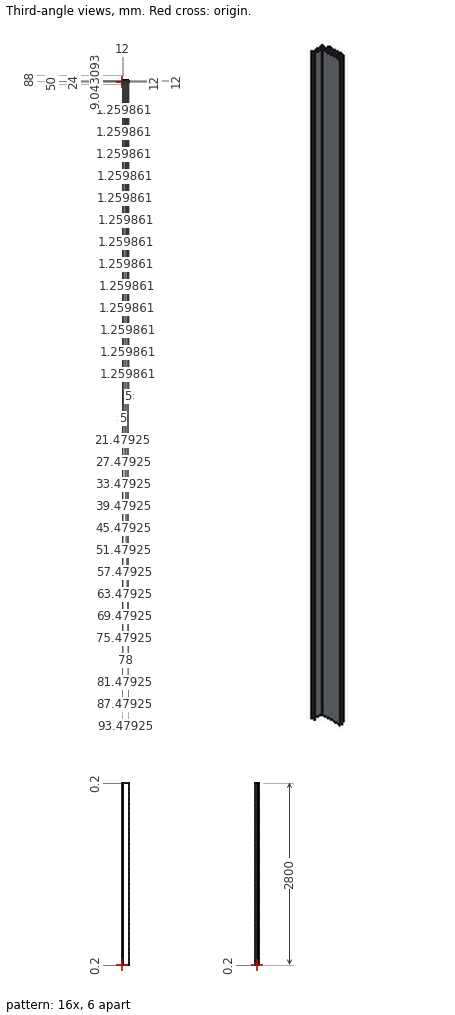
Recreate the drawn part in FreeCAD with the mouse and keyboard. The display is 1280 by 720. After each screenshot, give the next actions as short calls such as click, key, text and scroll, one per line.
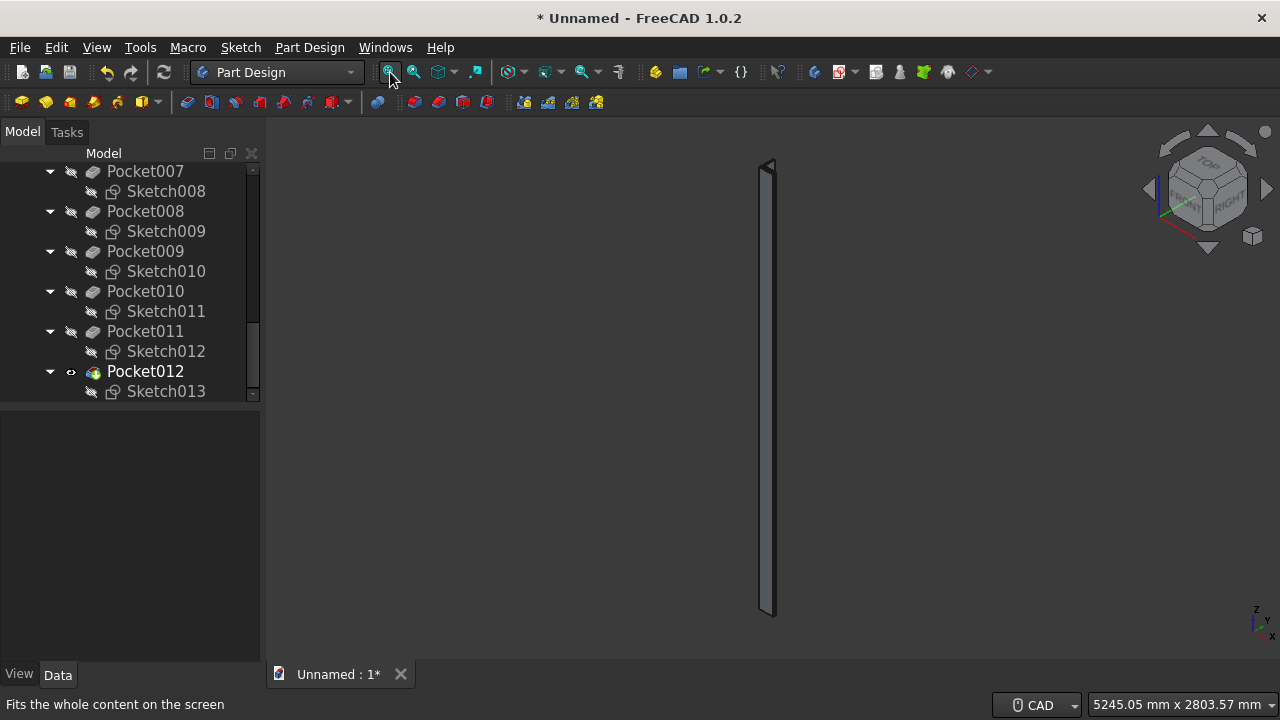
scroll(771, 172, up, 11)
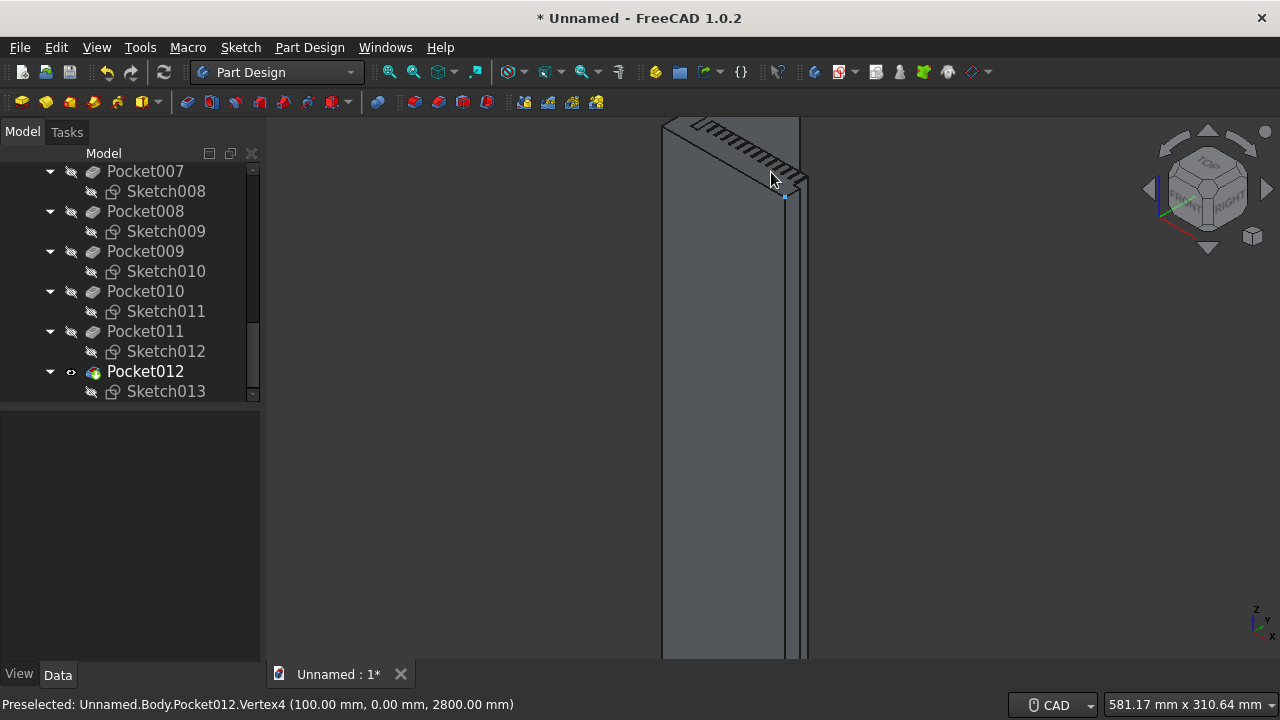
click(390, 72)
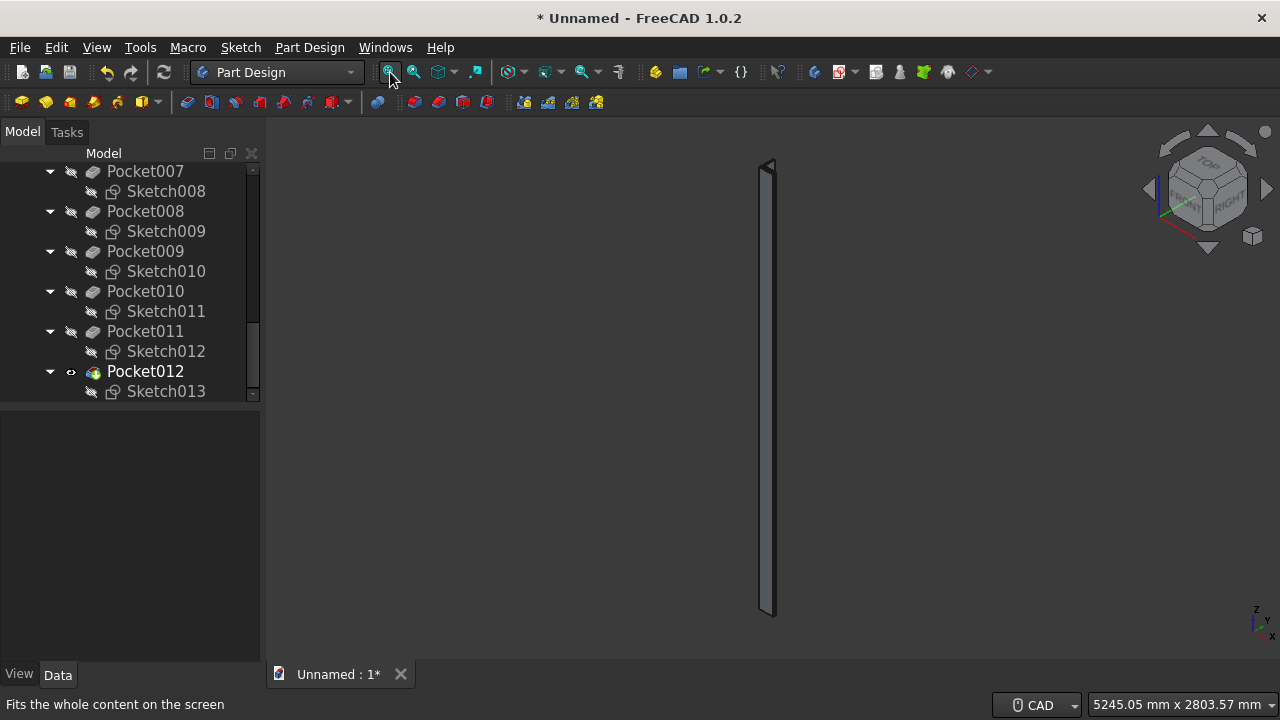
key(2)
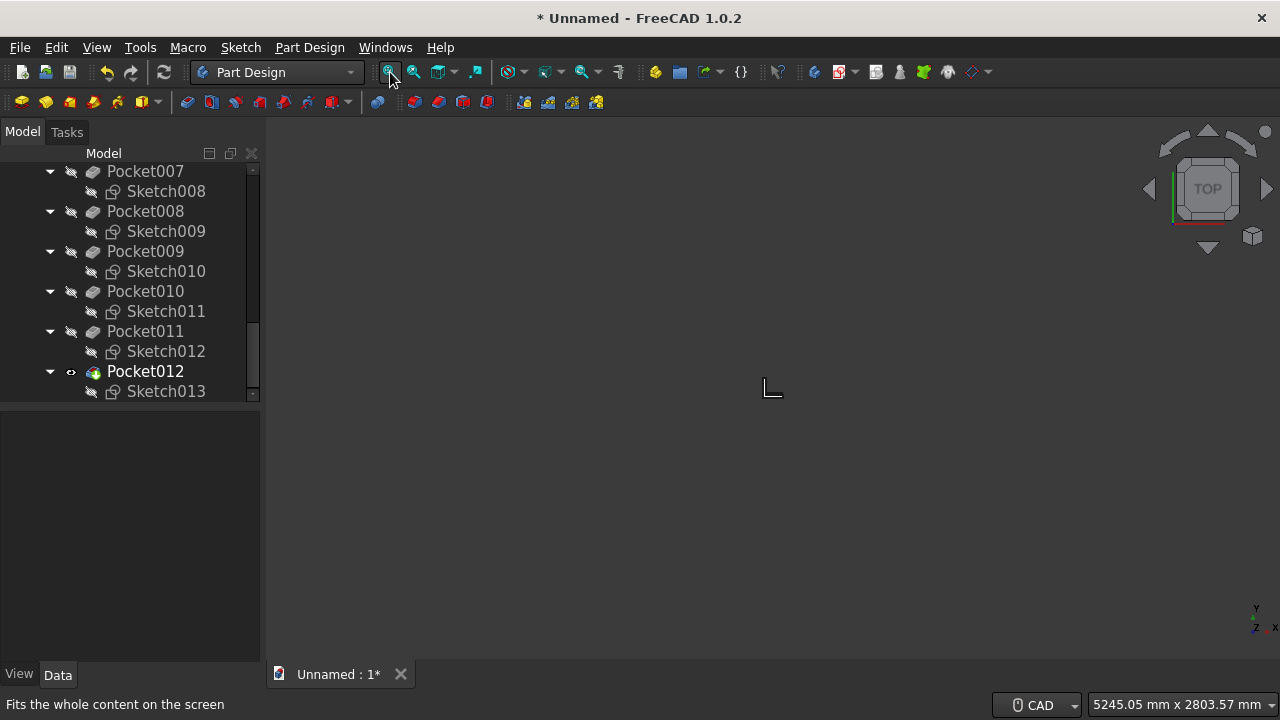
click(390, 72)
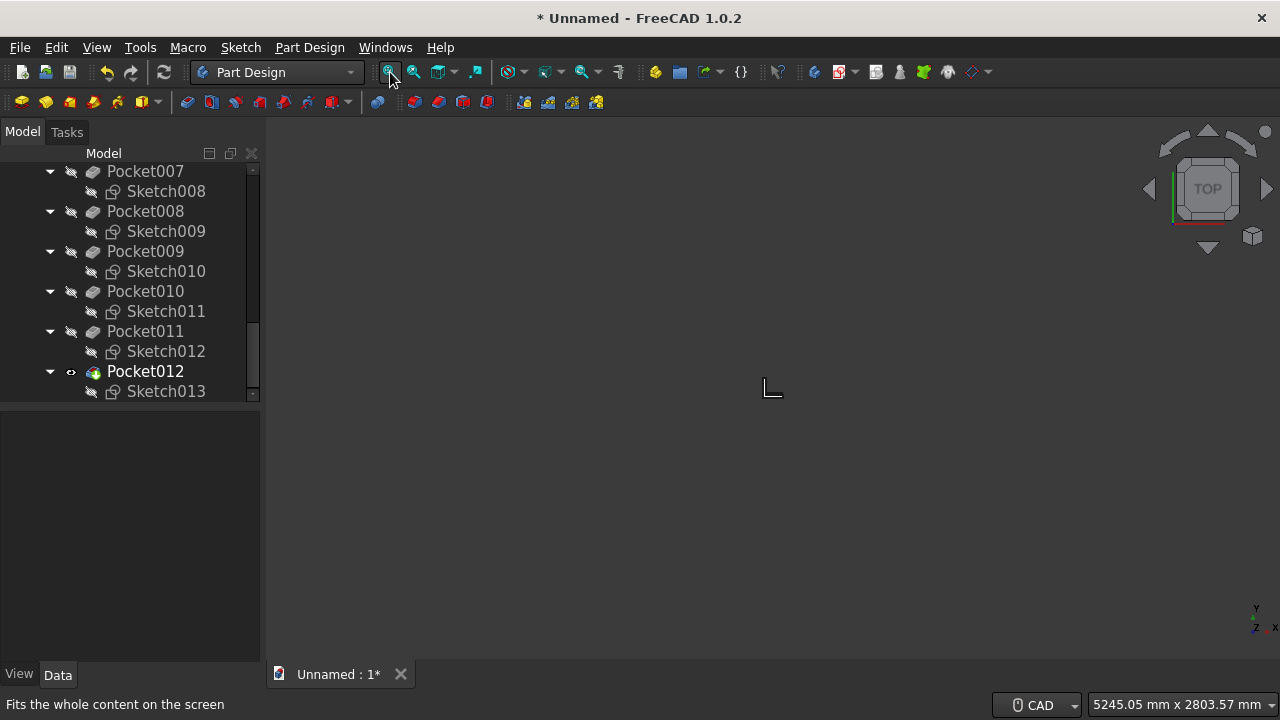
scroll(779, 395, up, 11)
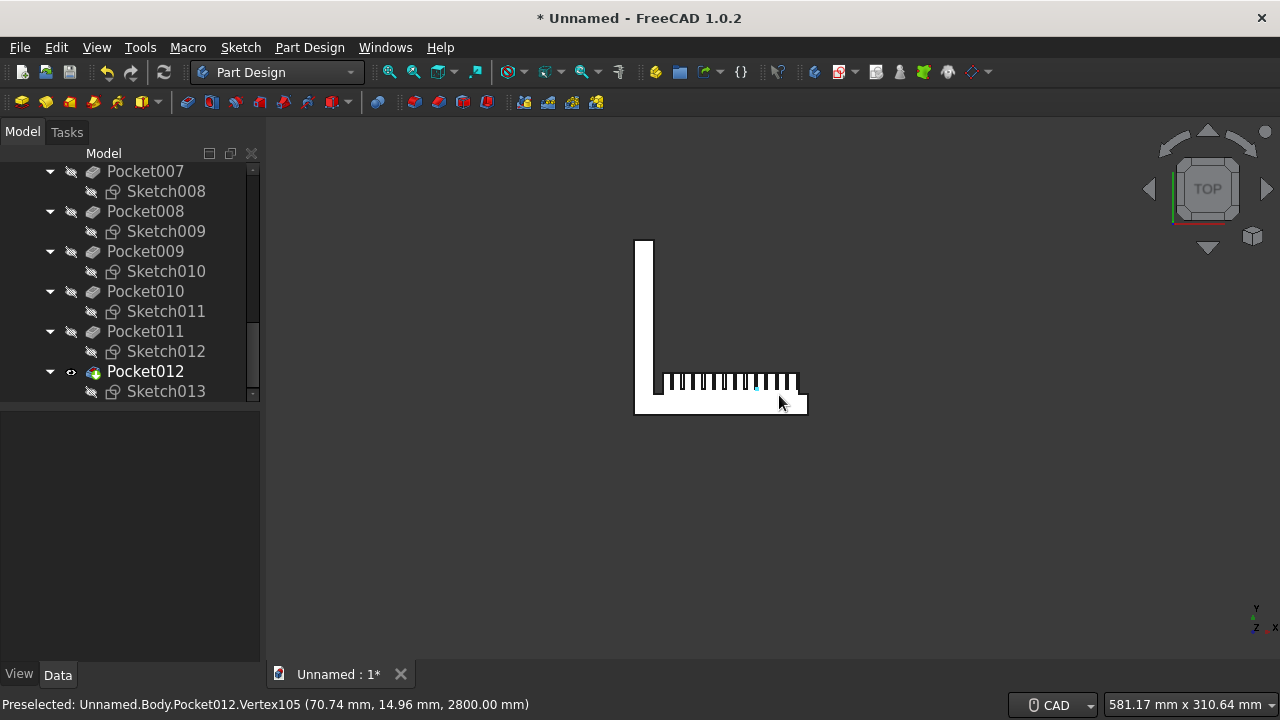
click(771, 401)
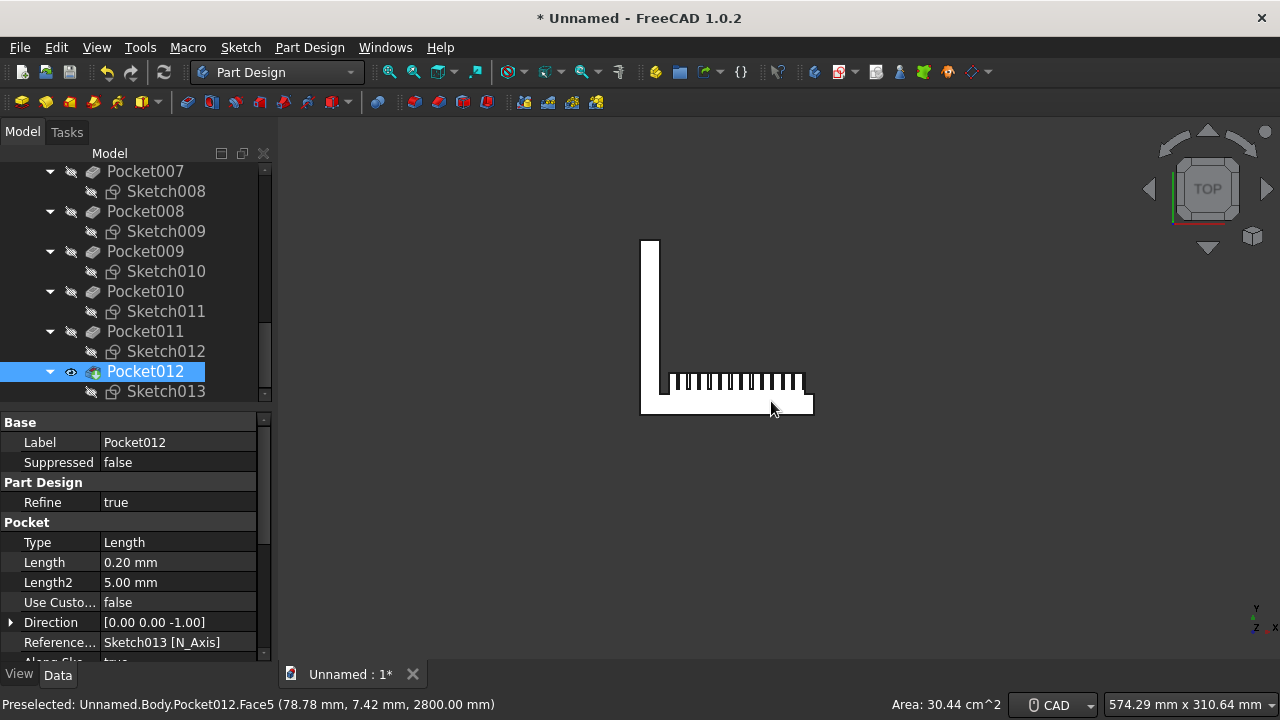
click(840, 72)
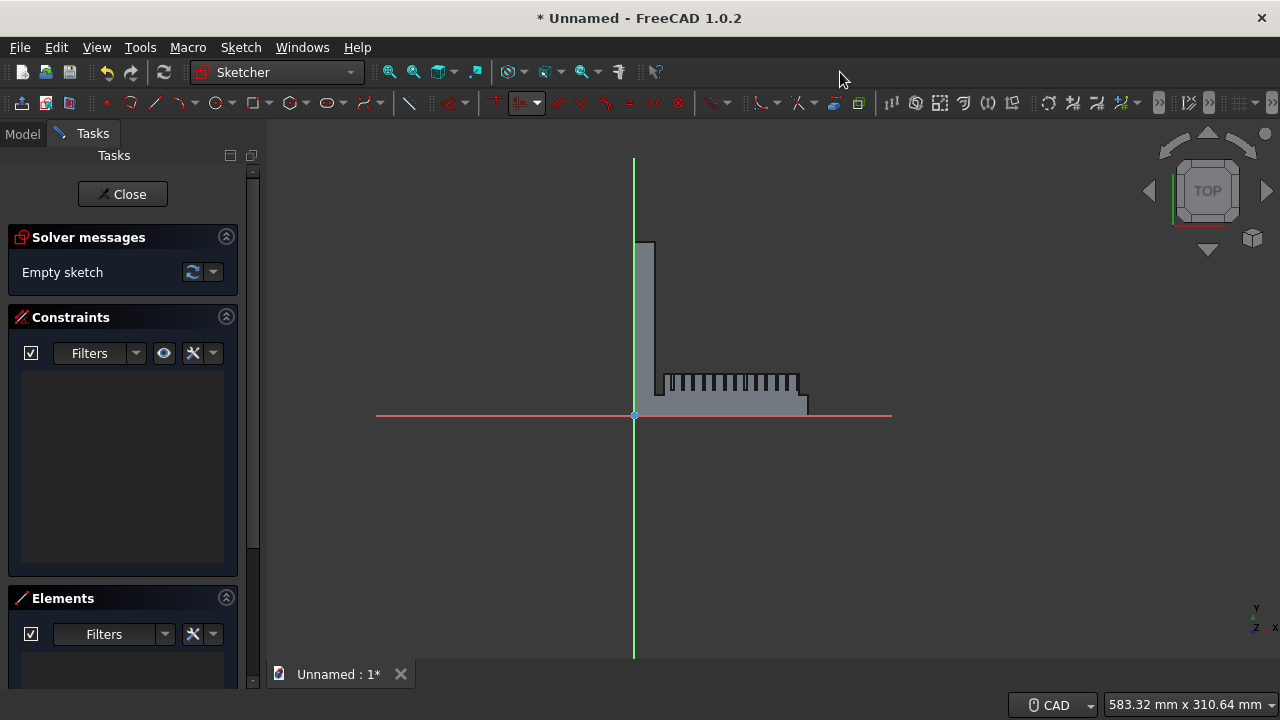
scroll(625, 455, up, 7)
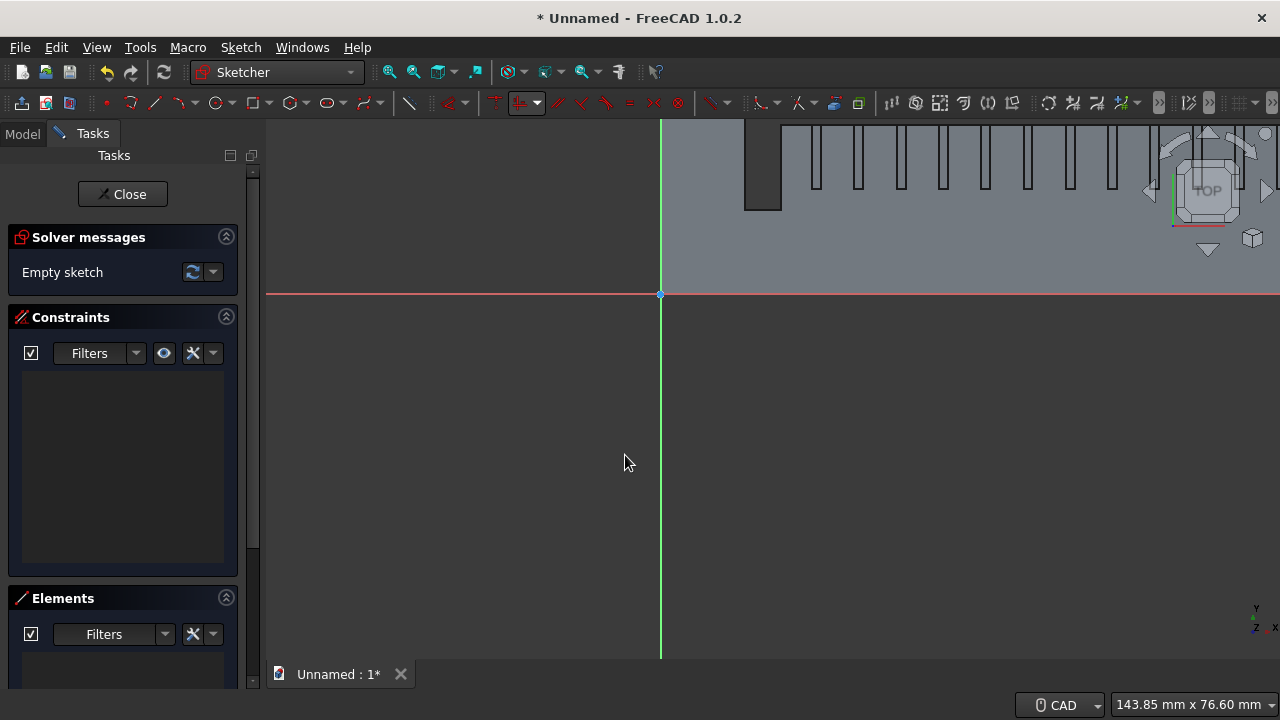
click(254, 104)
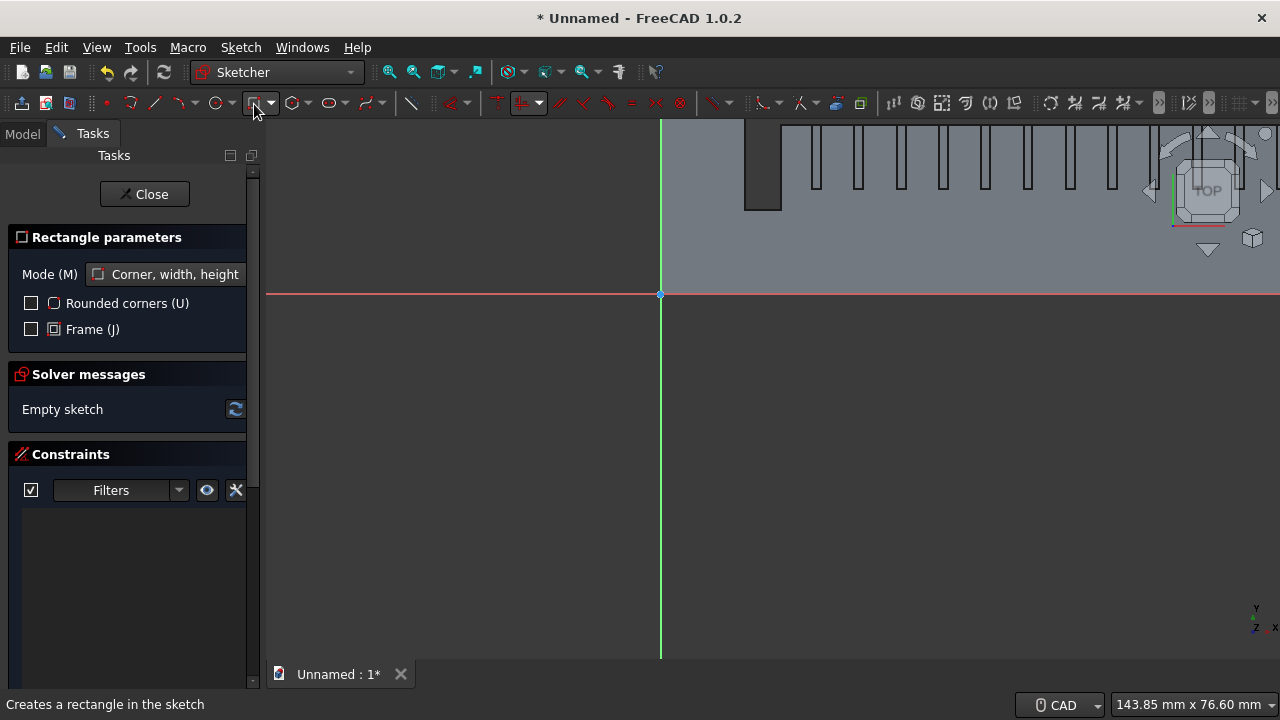
click(661, 210)
move(745, 562)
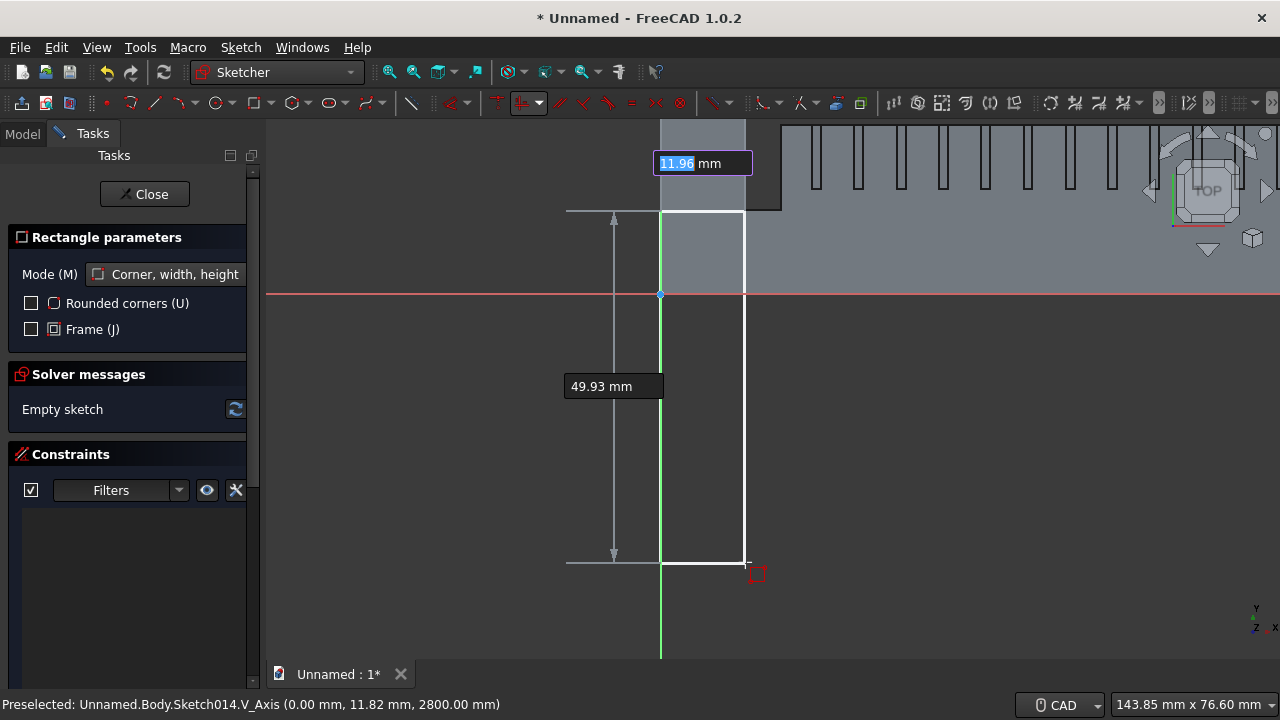
text(12)
key(Tab)
text(50)
key(Return)
key(Escape)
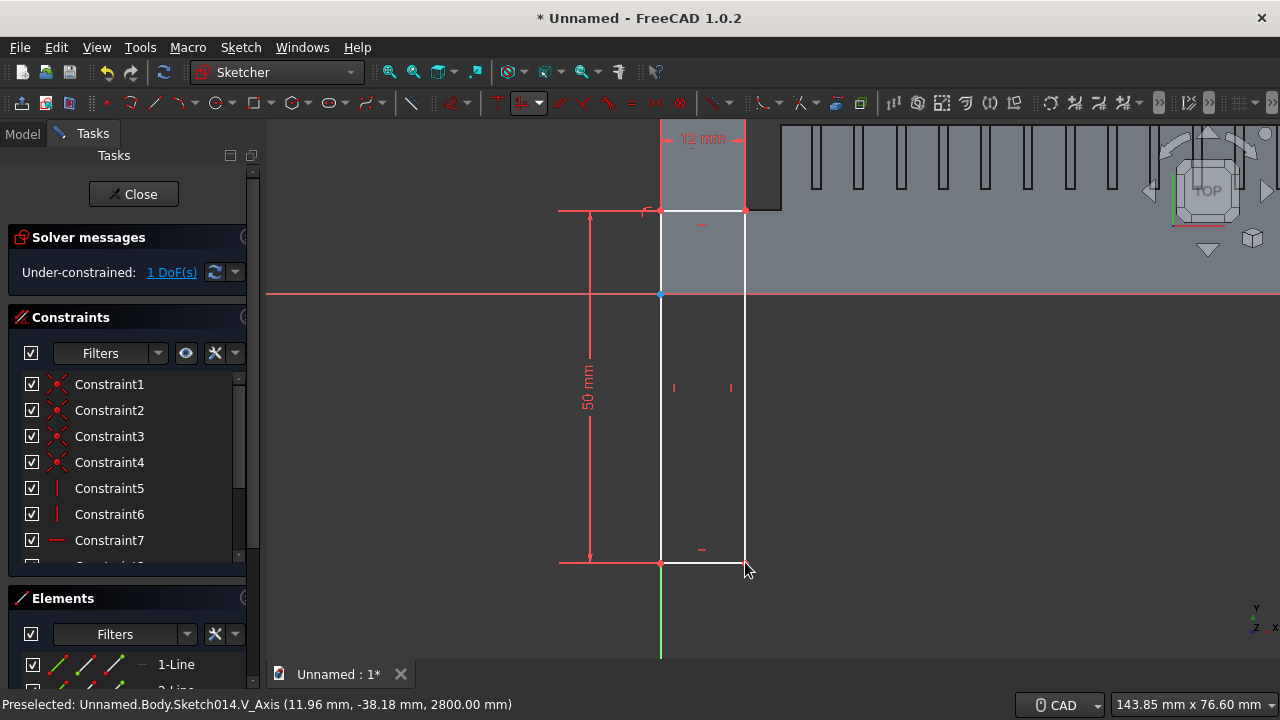
click(450, 104)